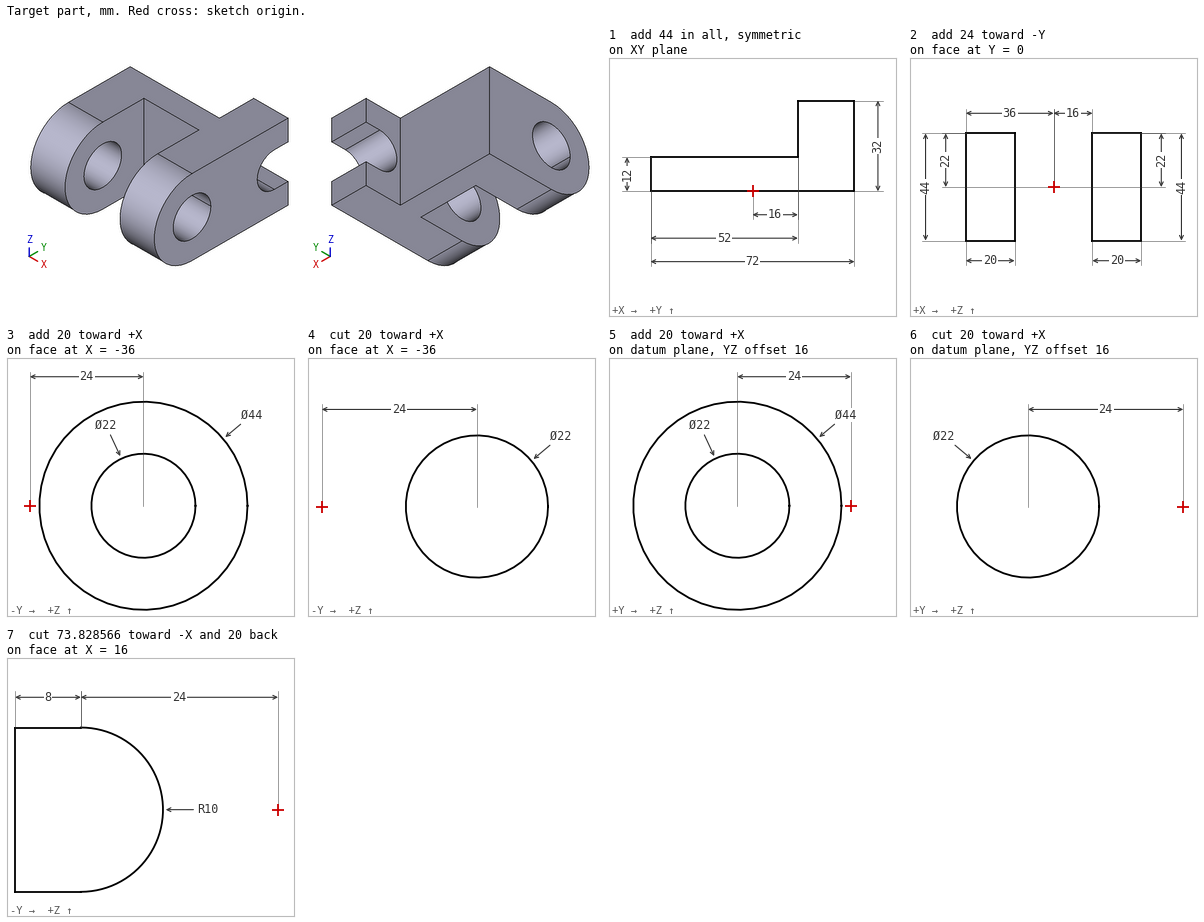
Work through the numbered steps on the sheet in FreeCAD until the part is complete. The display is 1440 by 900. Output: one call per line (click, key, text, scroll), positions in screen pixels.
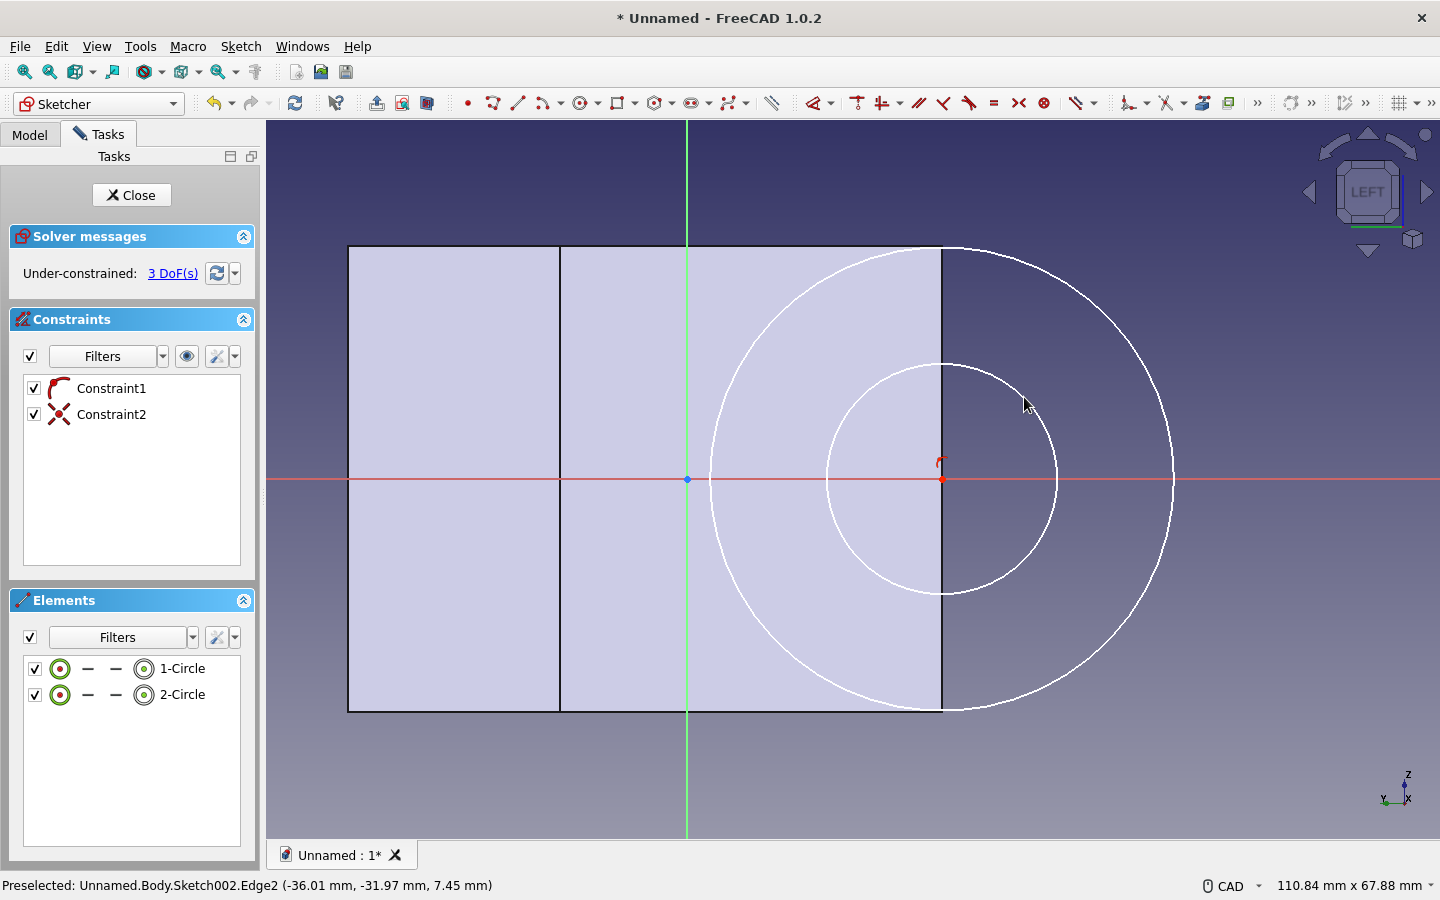
click(812, 104)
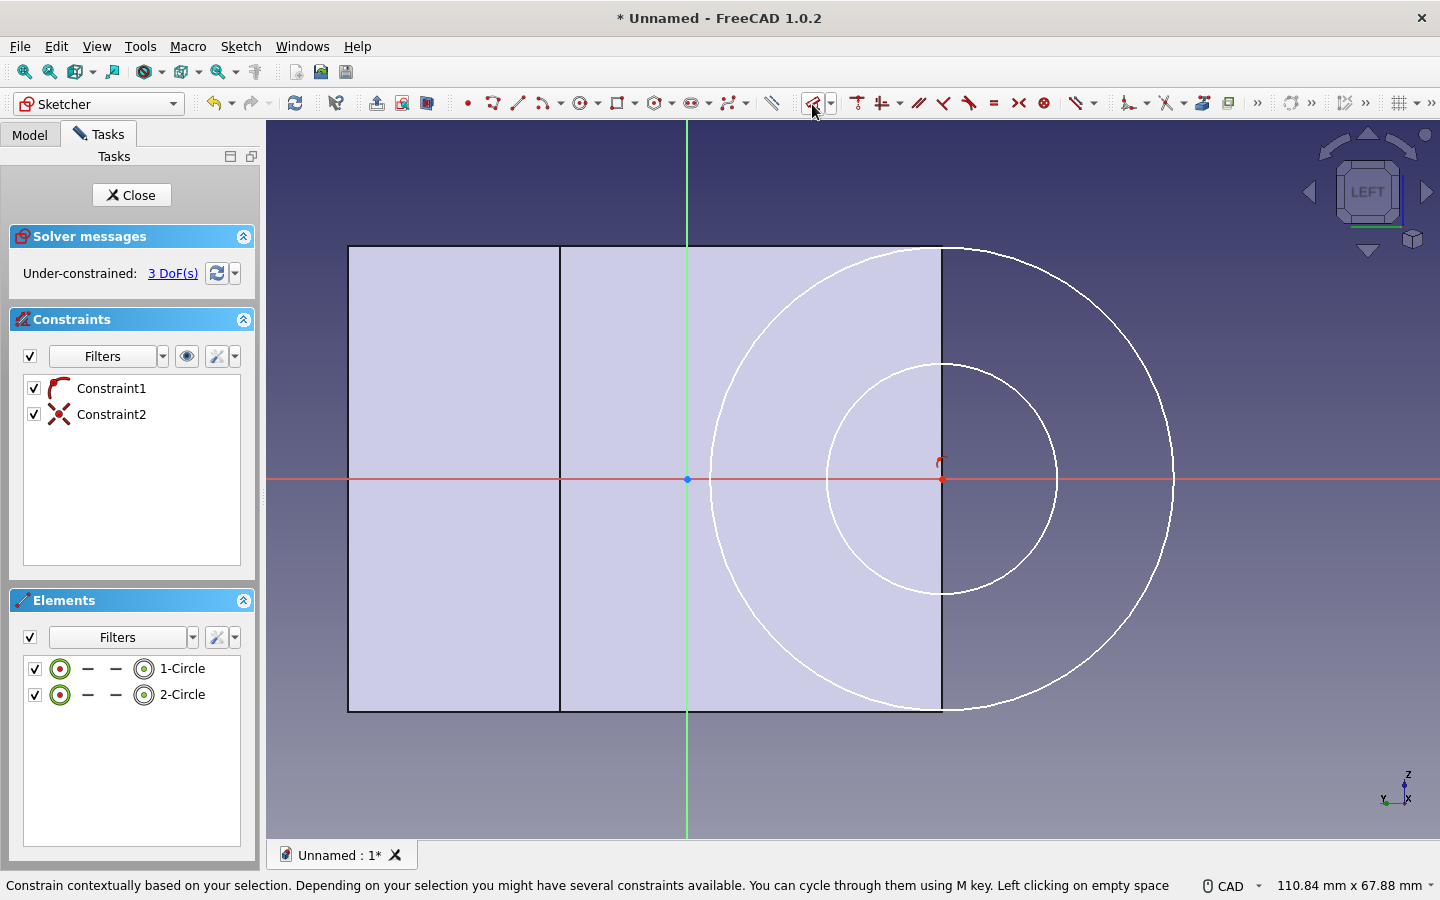
click(1105, 314)
click(1127, 291)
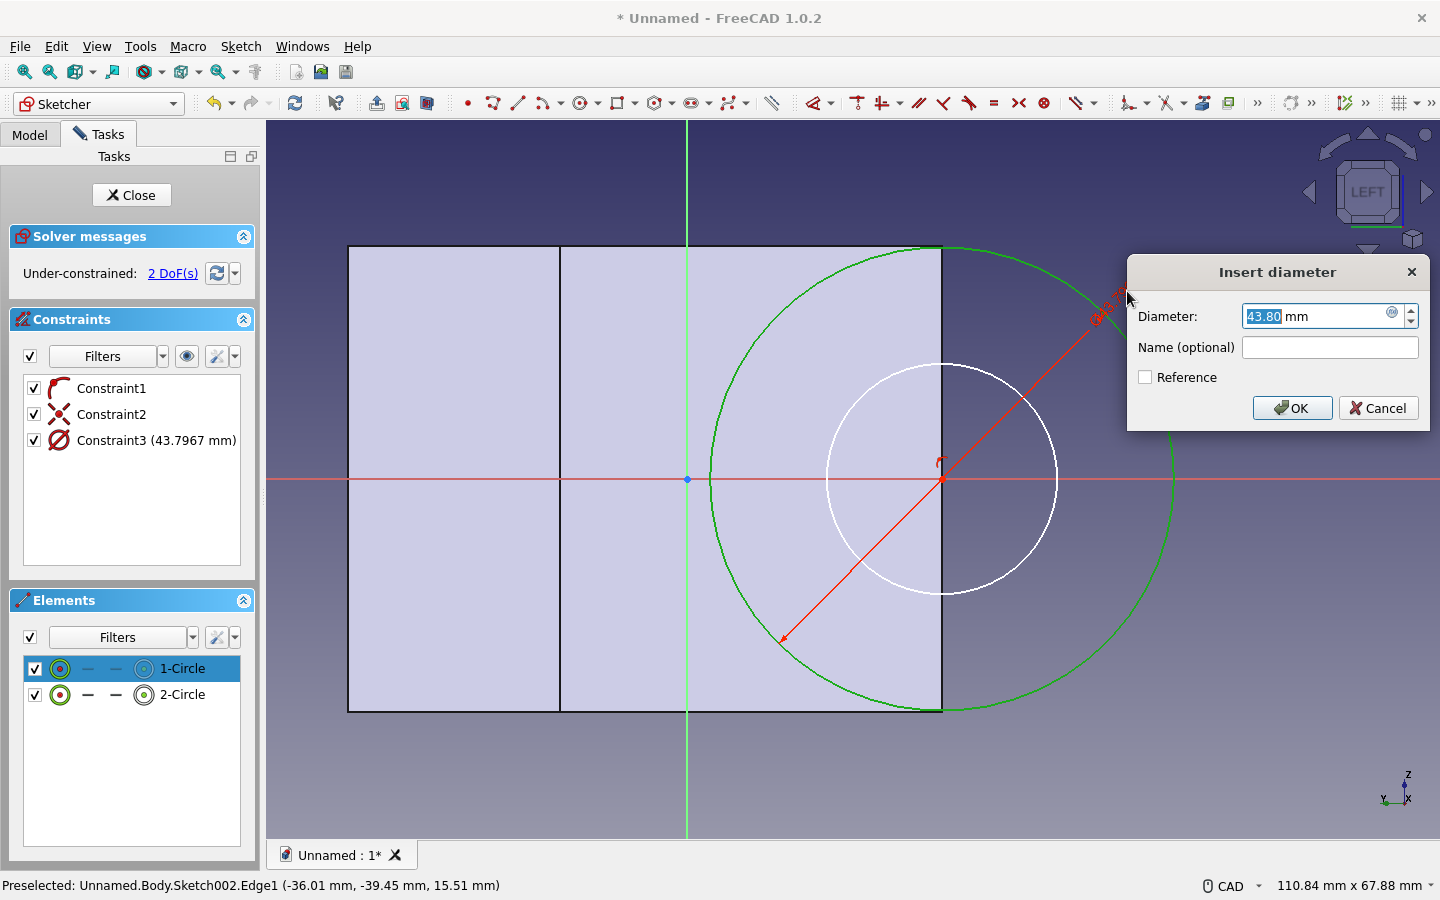
text(44)
key(Return)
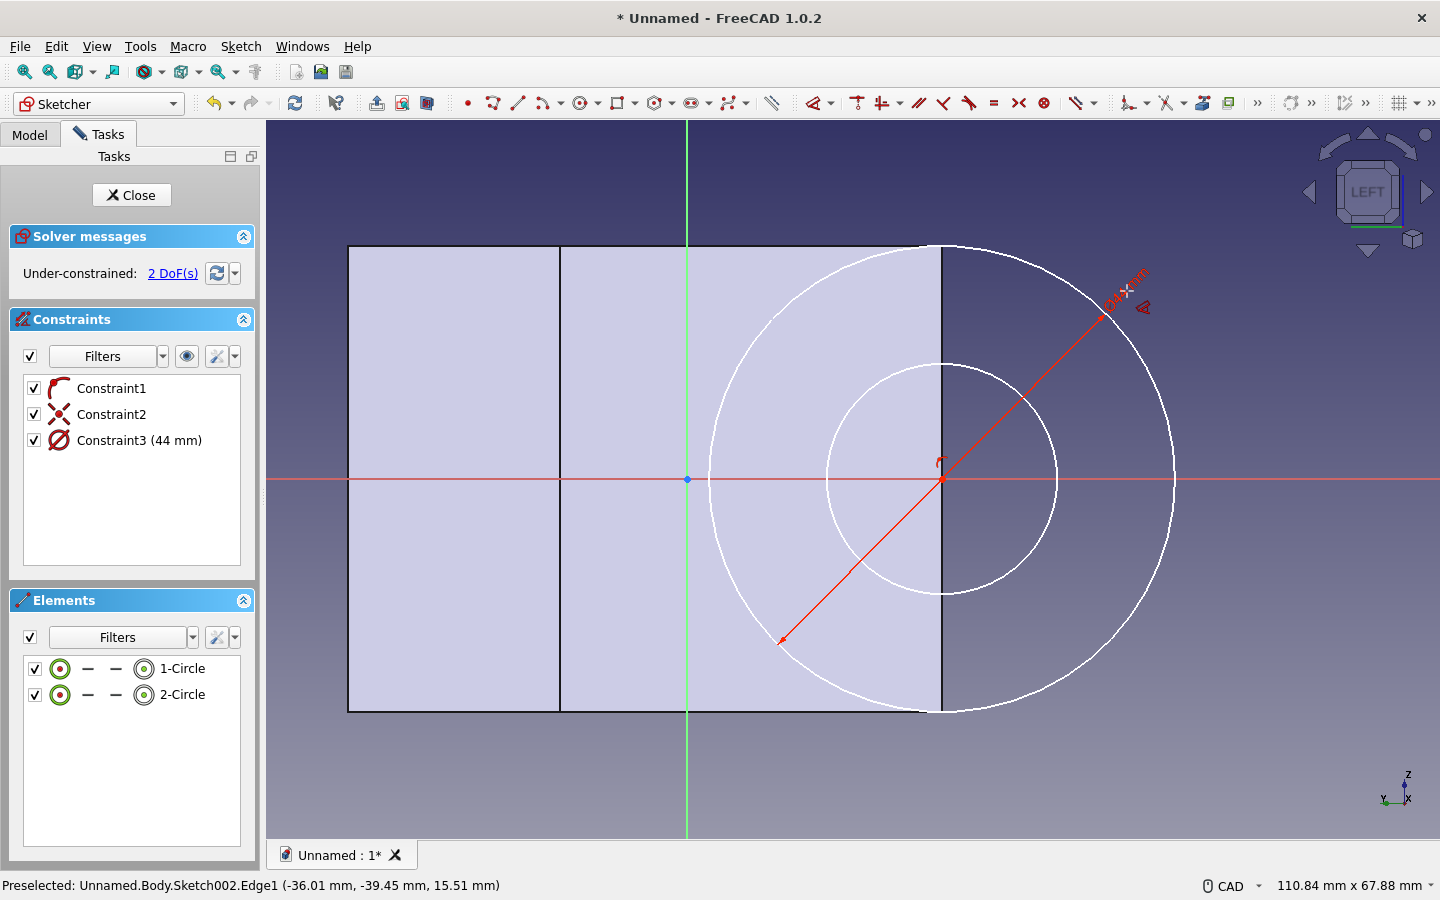
click(1023, 397)
click(1045, 374)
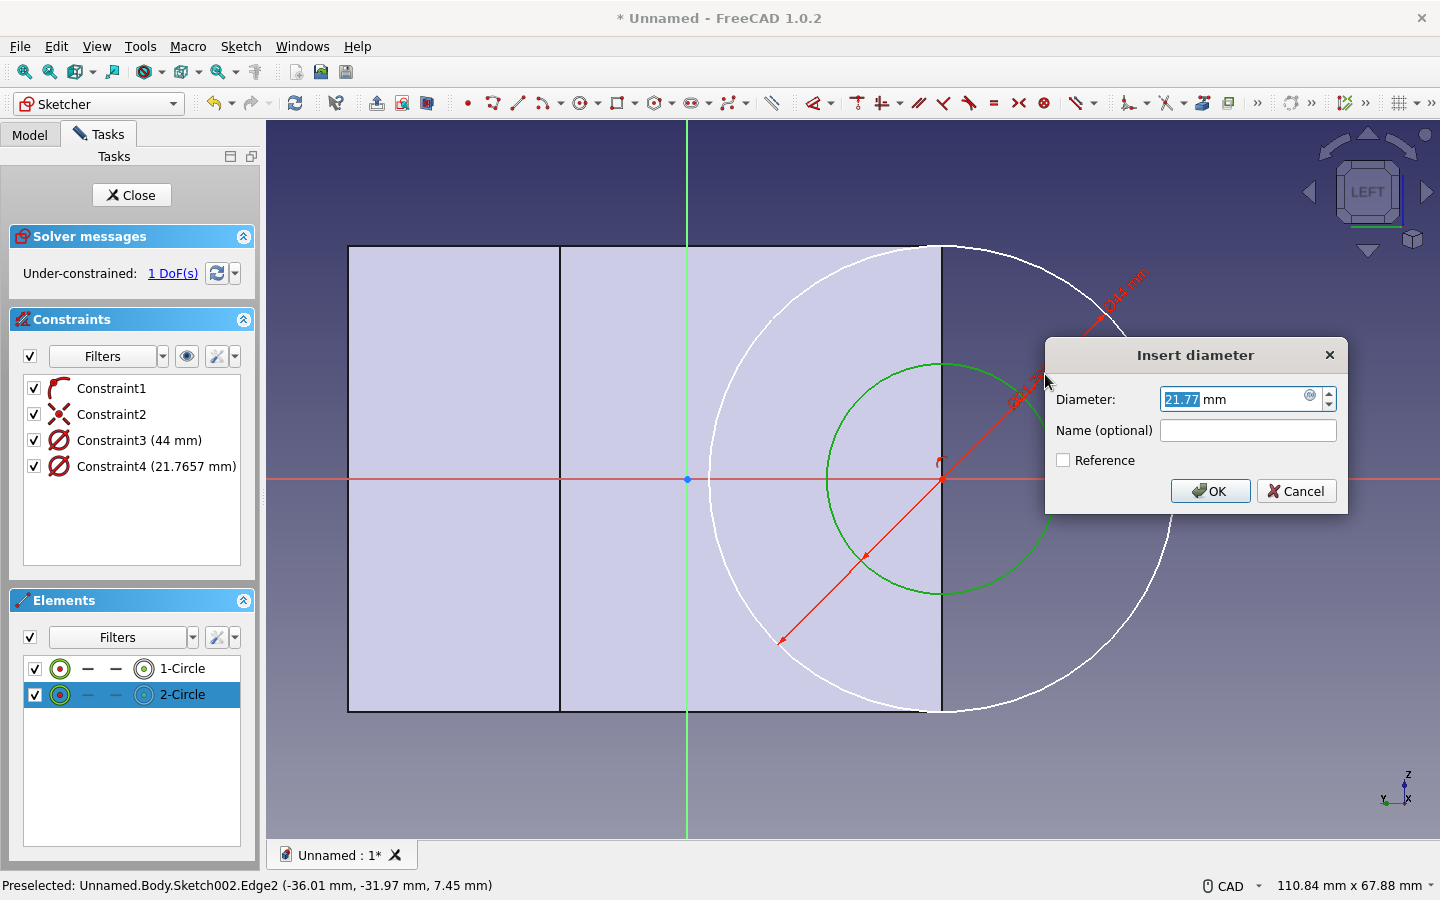
text(22)
key(Return)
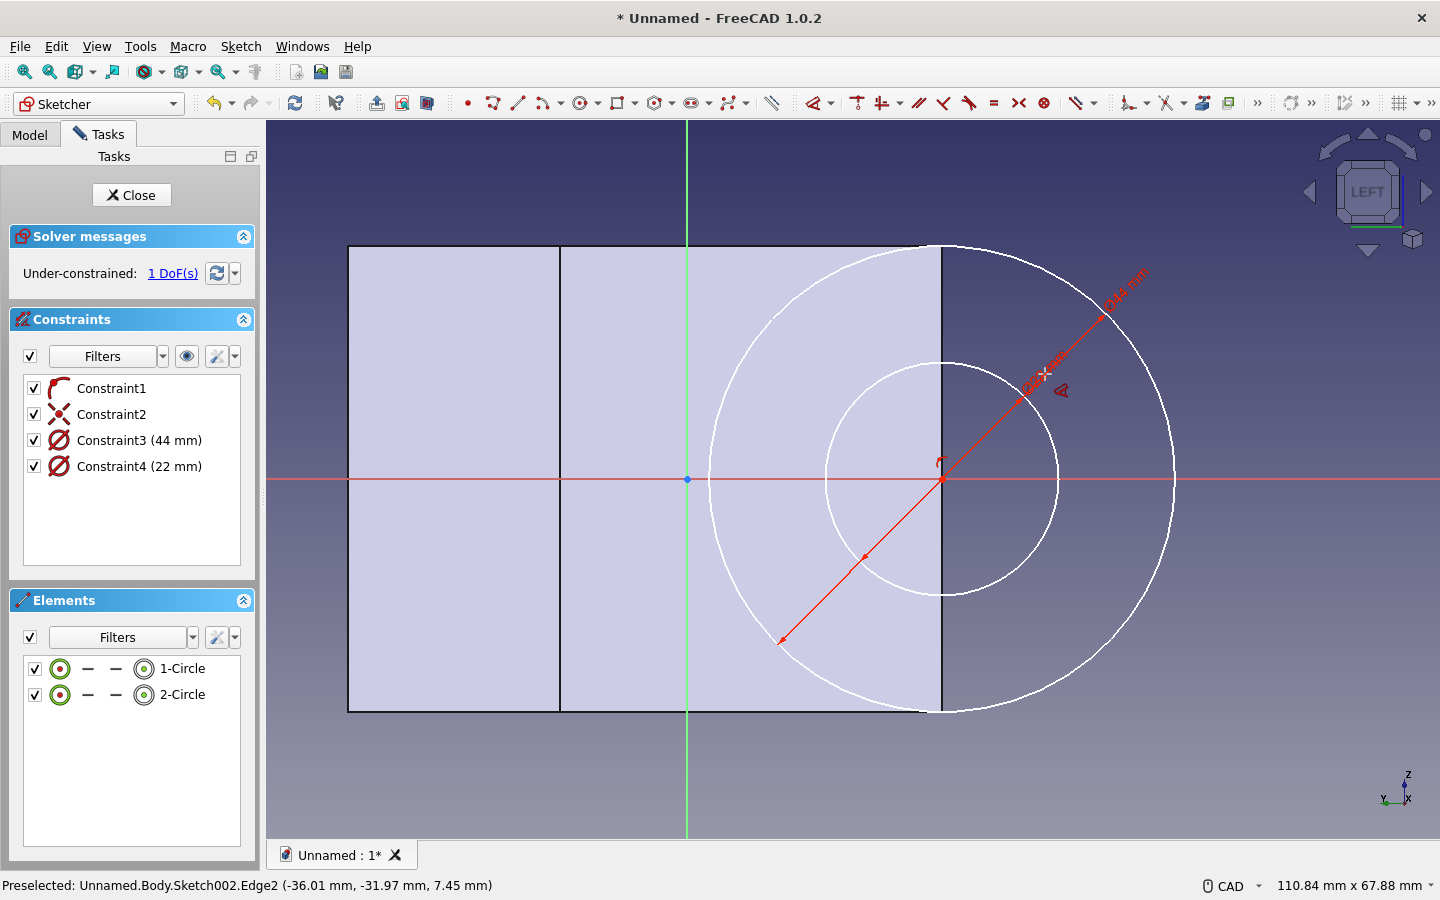
click(942, 479)
click(815, 513)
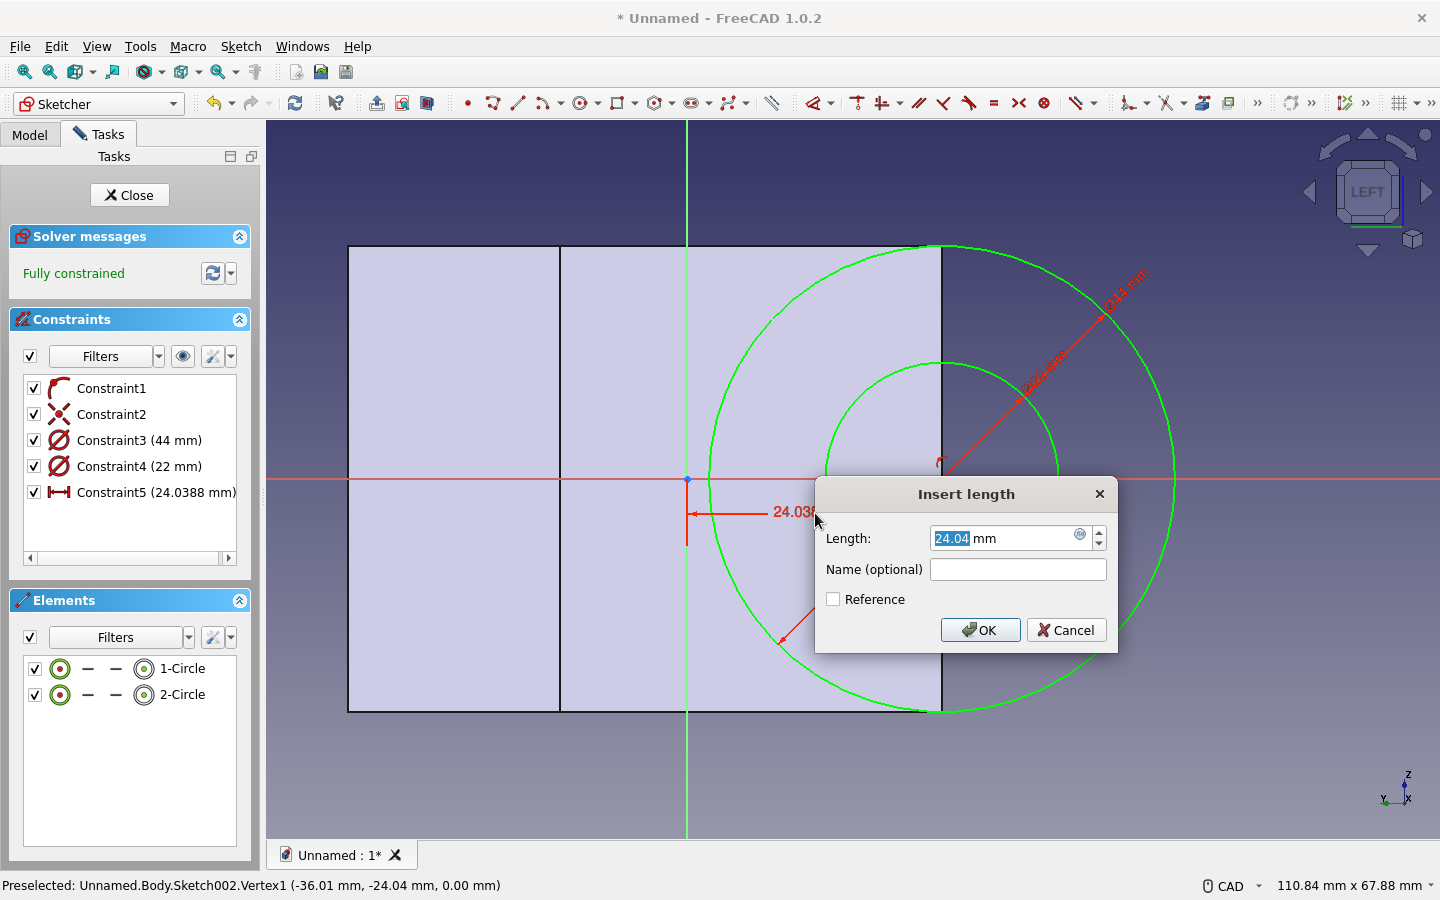
text(24)
key(Return)
key(Escape)